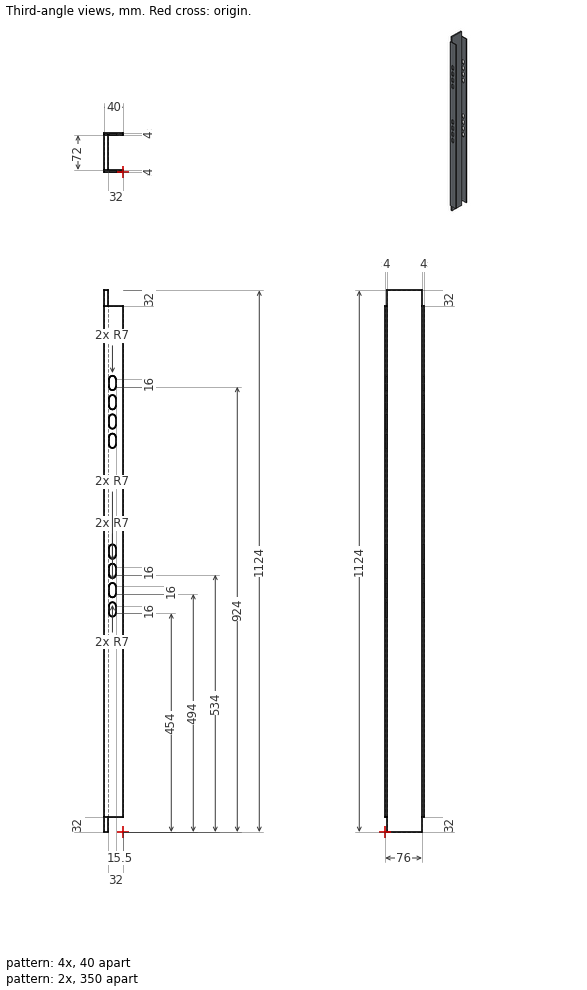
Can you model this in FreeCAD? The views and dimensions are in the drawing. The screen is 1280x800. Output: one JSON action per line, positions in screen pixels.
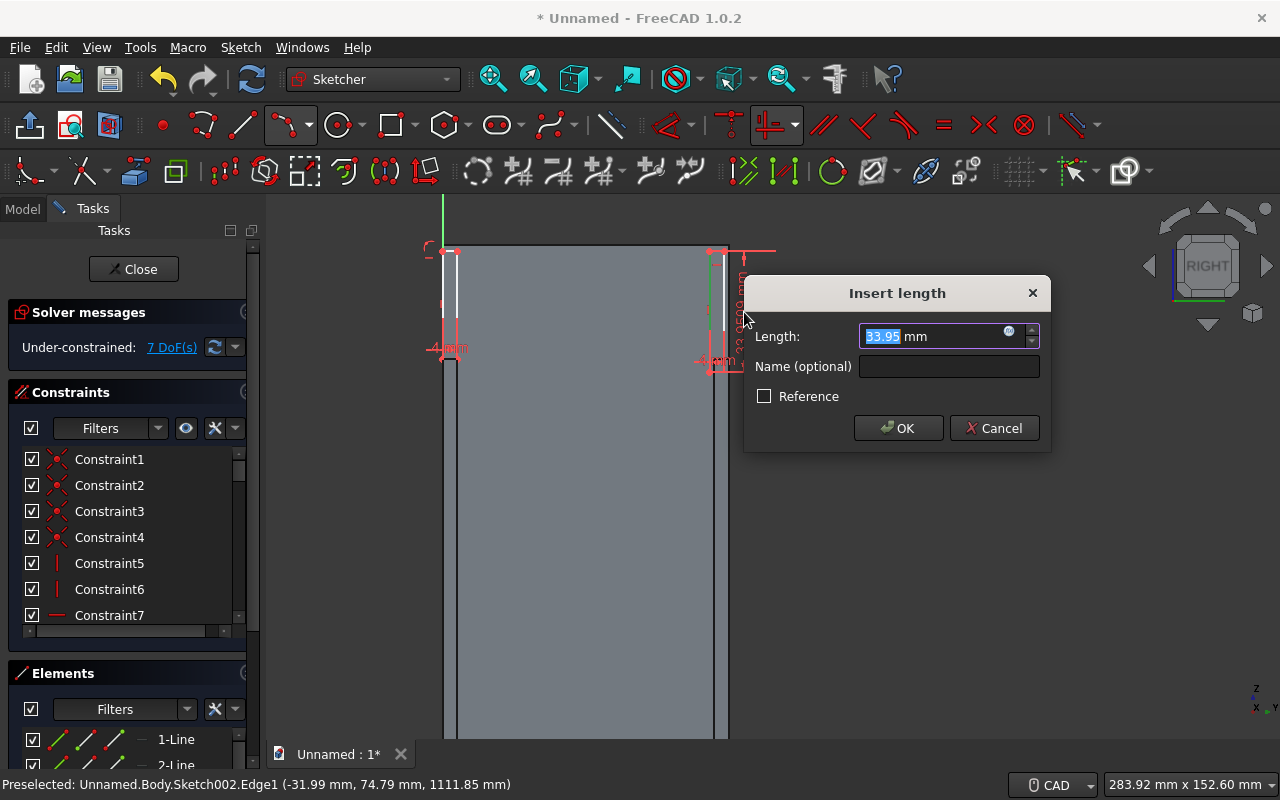
{"action": "type", "text": "32"}
{"action": "key", "text": "Return"}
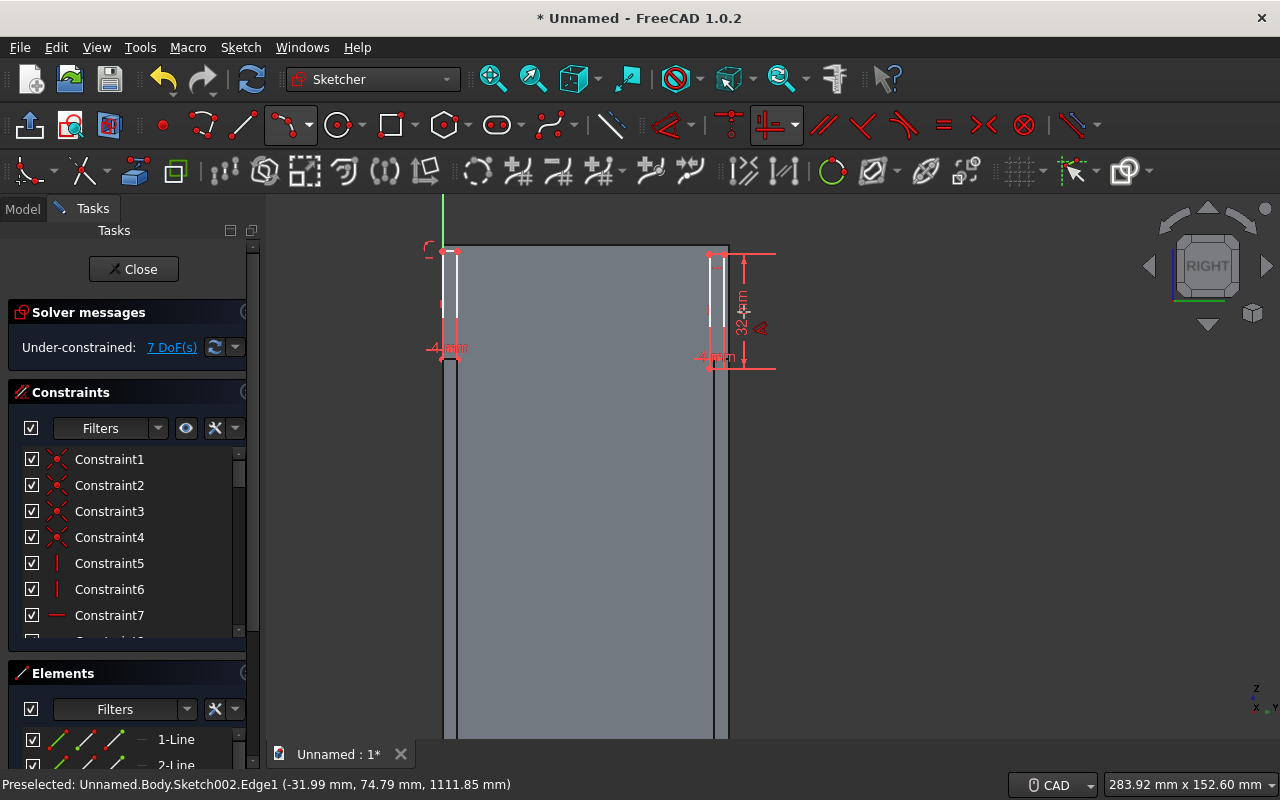
{"action": "left_click", "coordinate": [443, 284]}
{"action": "left_click", "coordinate": [409, 305]}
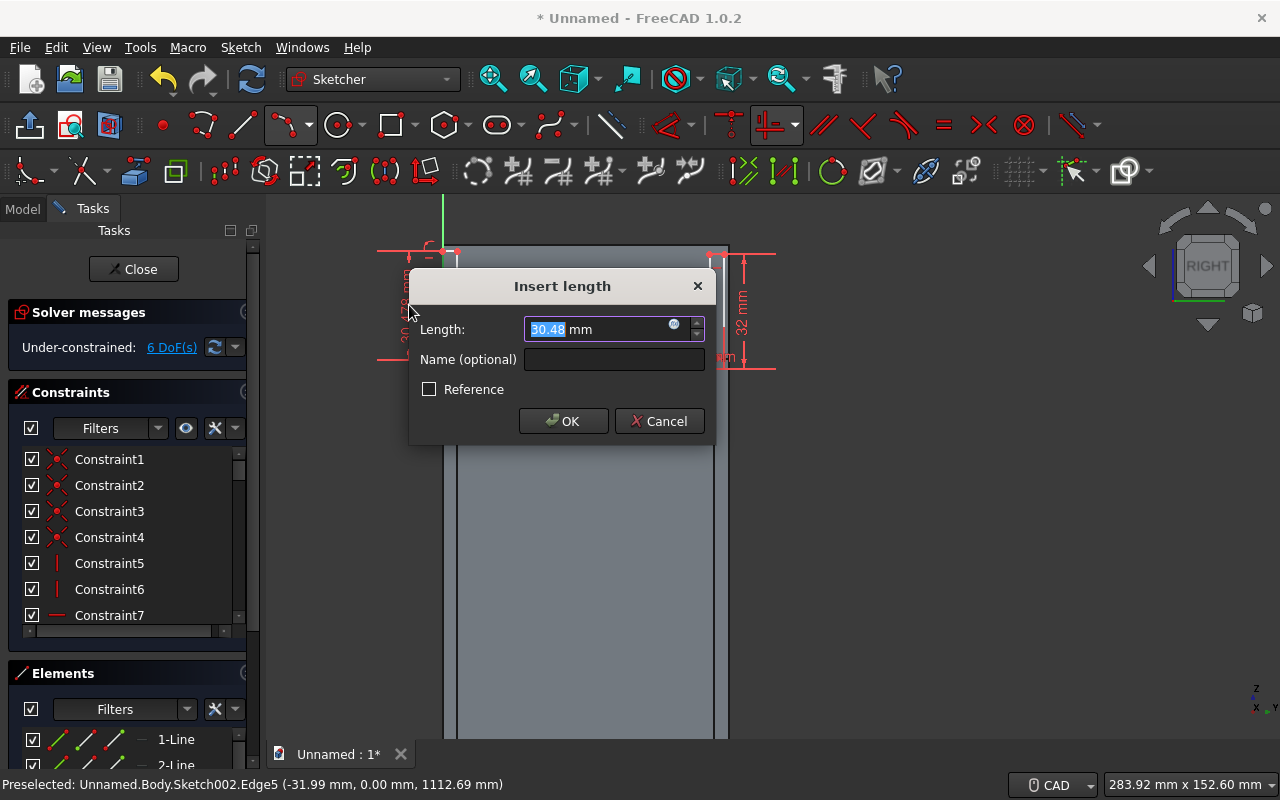
{"action": "type", "text": "32"}
{"action": "key", "text": "Return"}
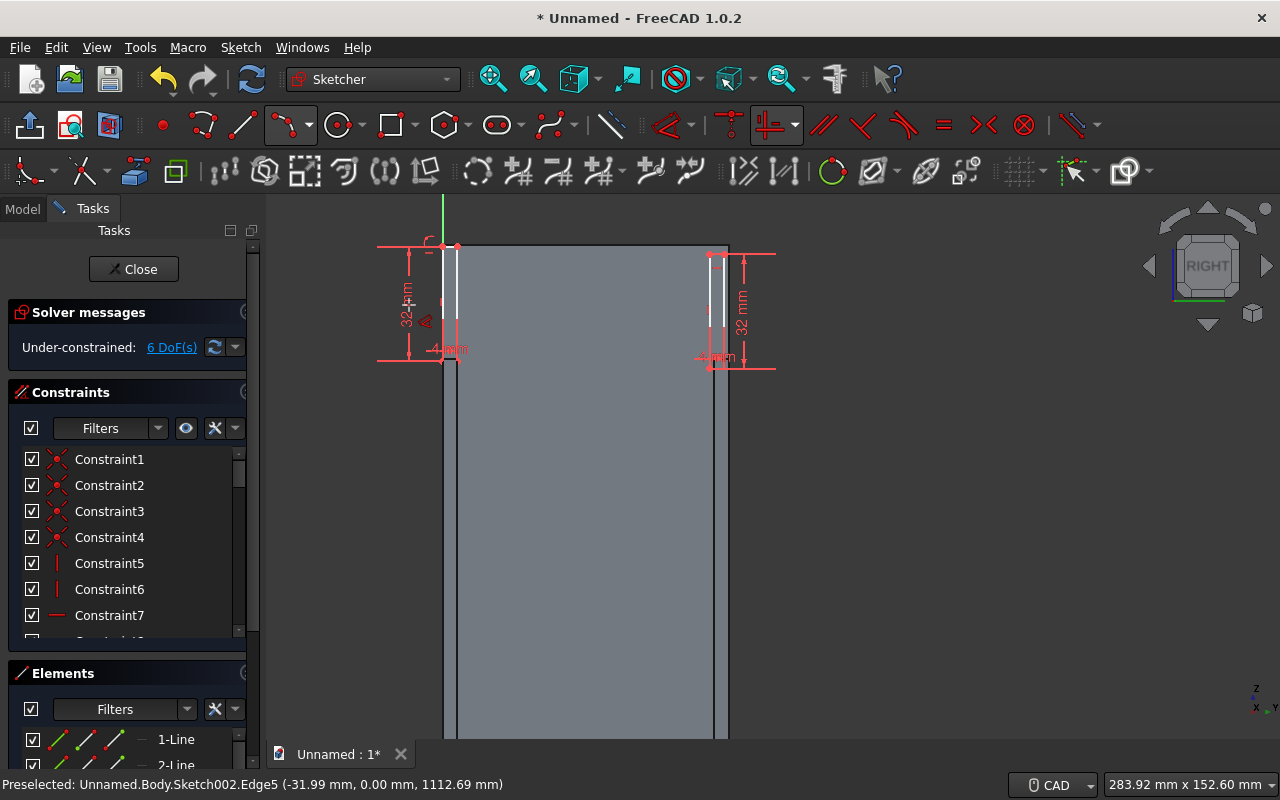
{"action": "scroll", "coordinate": [716, 288], "scroll_direction": "down", "scroll_amount": 12}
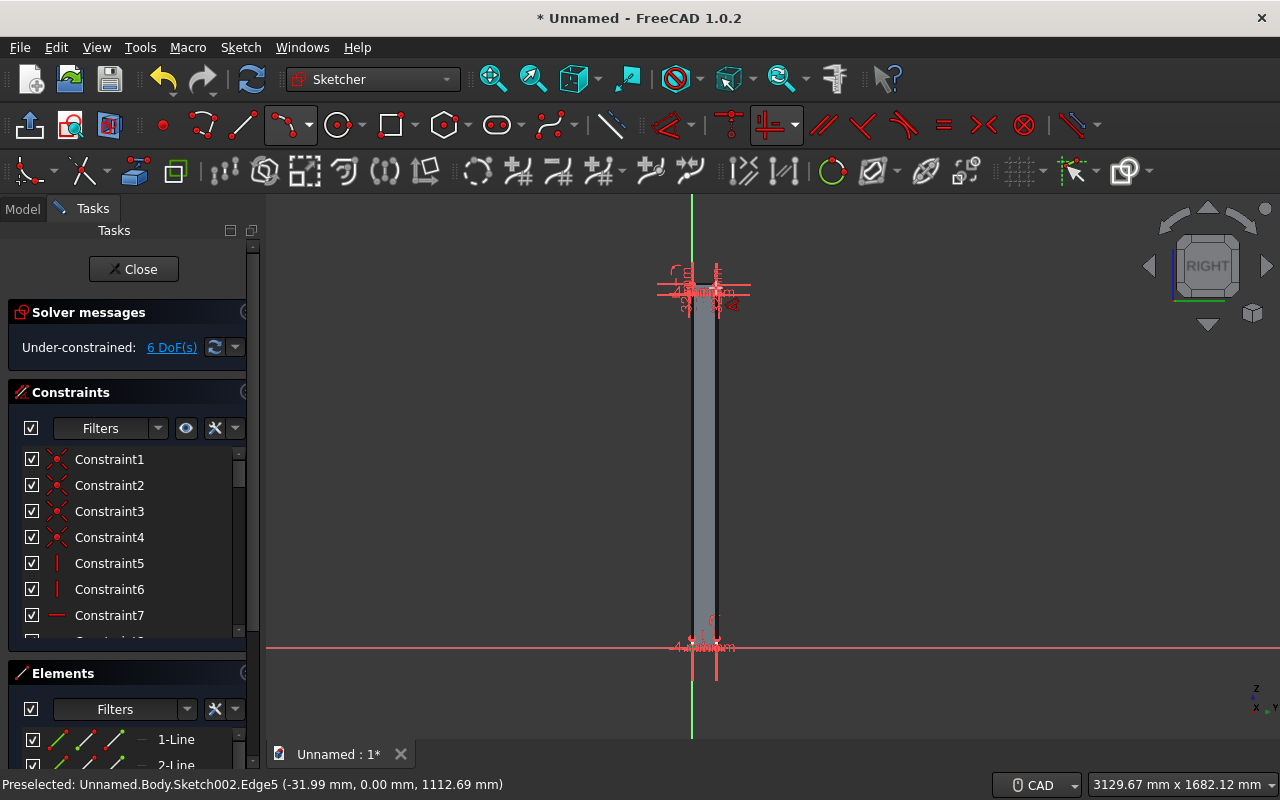
{"action": "scroll", "coordinate": [716, 642], "scroll_direction": "up", "scroll_amount": 12}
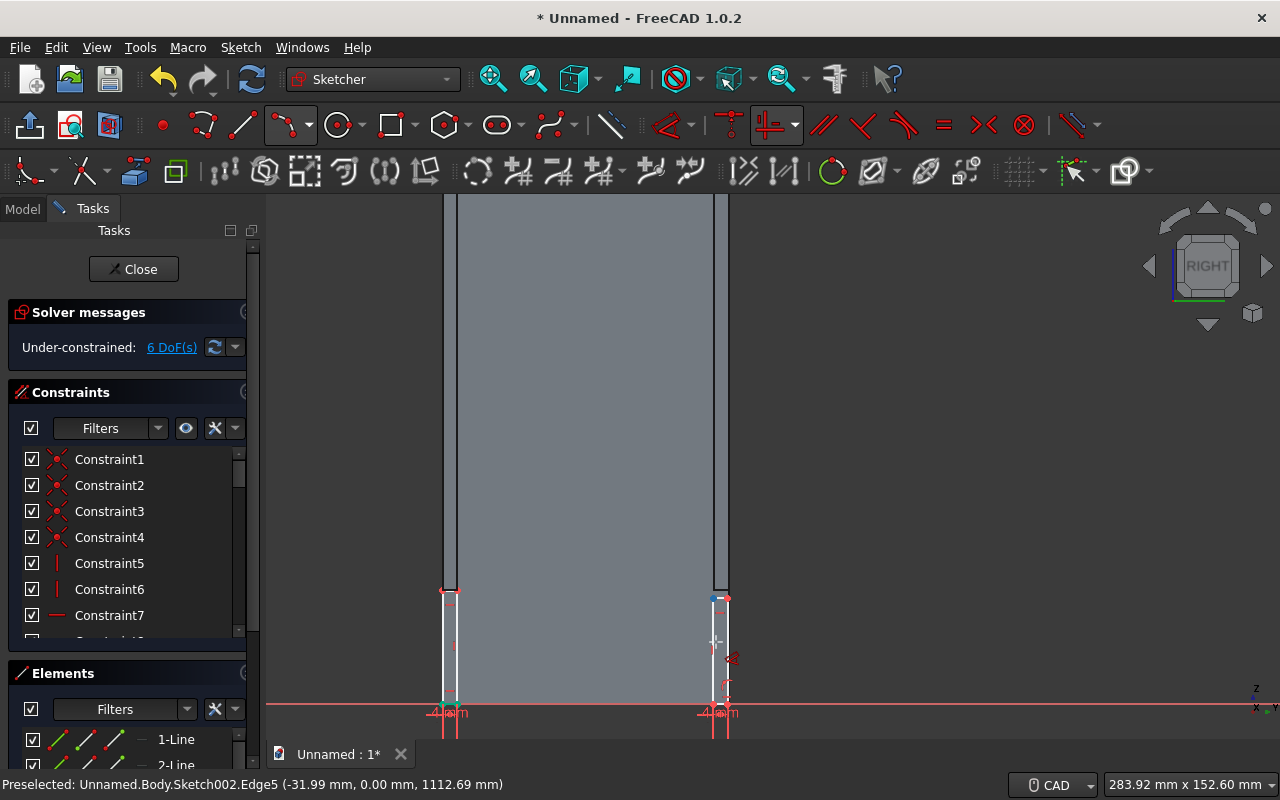
{"action": "left_click", "coordinate": [713, 630]}
{"action": "left_click", "coordinate": [747, 651]}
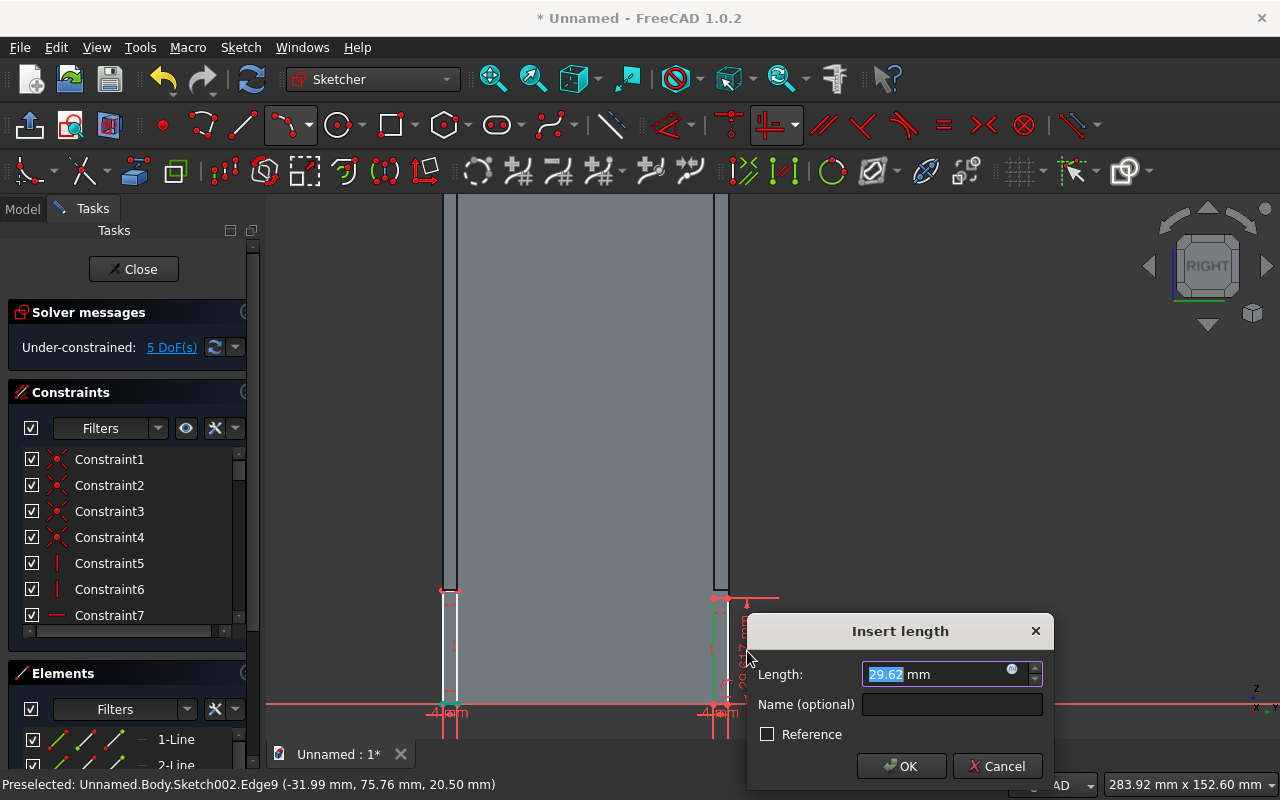
{"action": "type", "text": "32"}
{"action": "key", "text": "Return"}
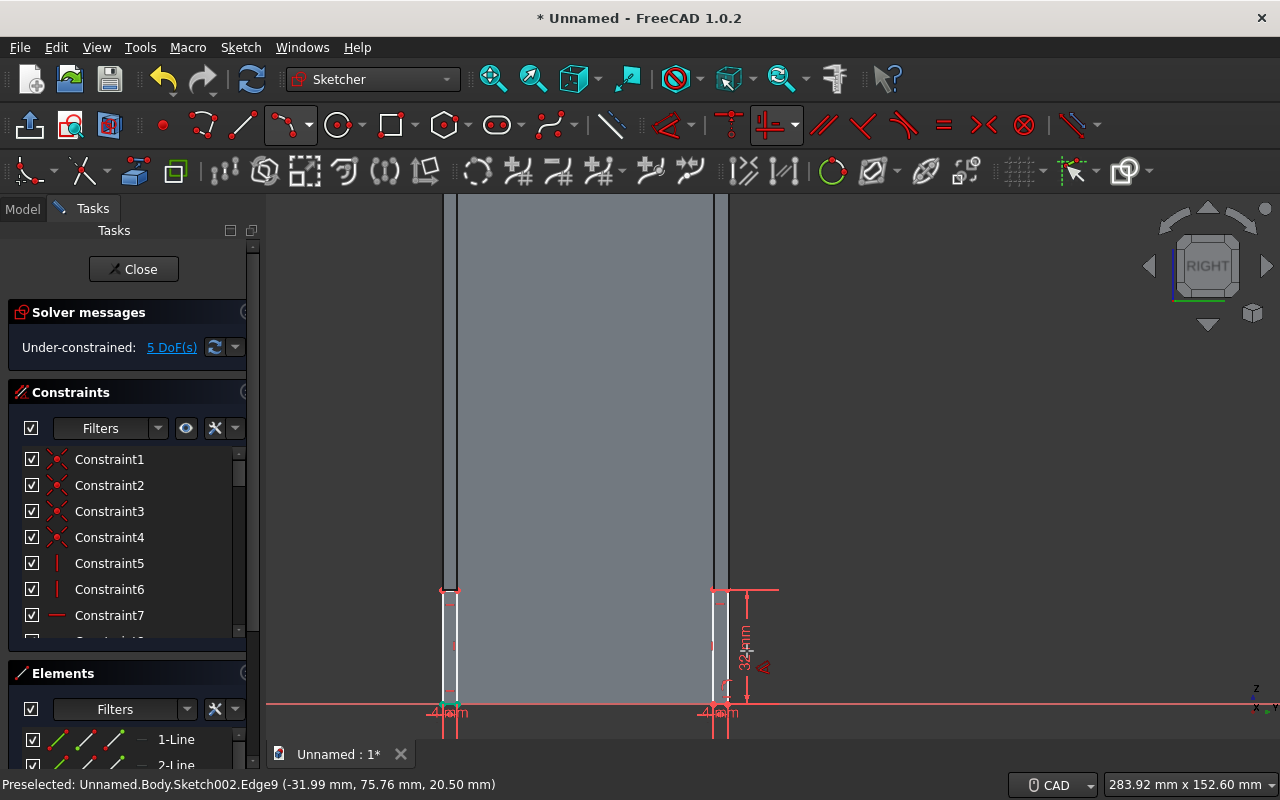
{"action": "left_click", "coordinate": [457, 670]}
{"action": "left_click", "coordinate": [423, 647]}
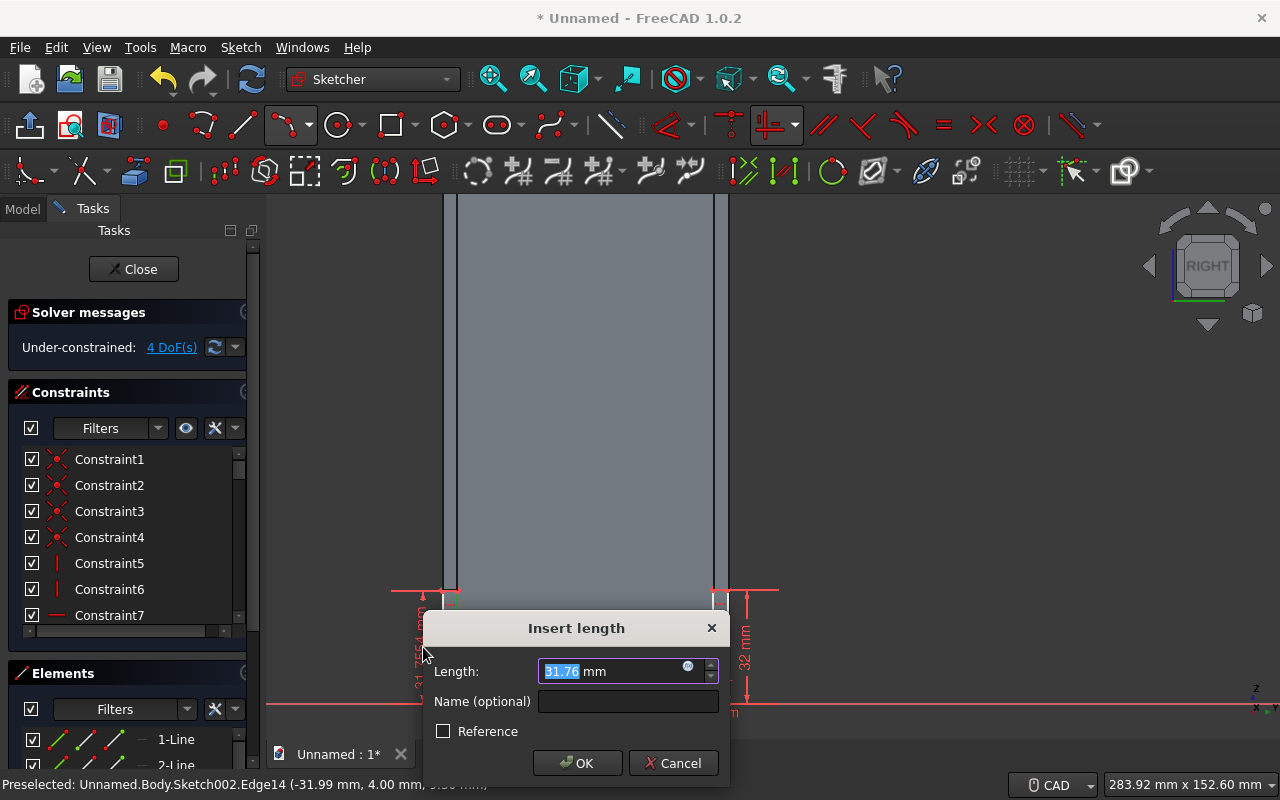
{"action": "type", "text": "32"}
{"action": "key", "text": "Return"}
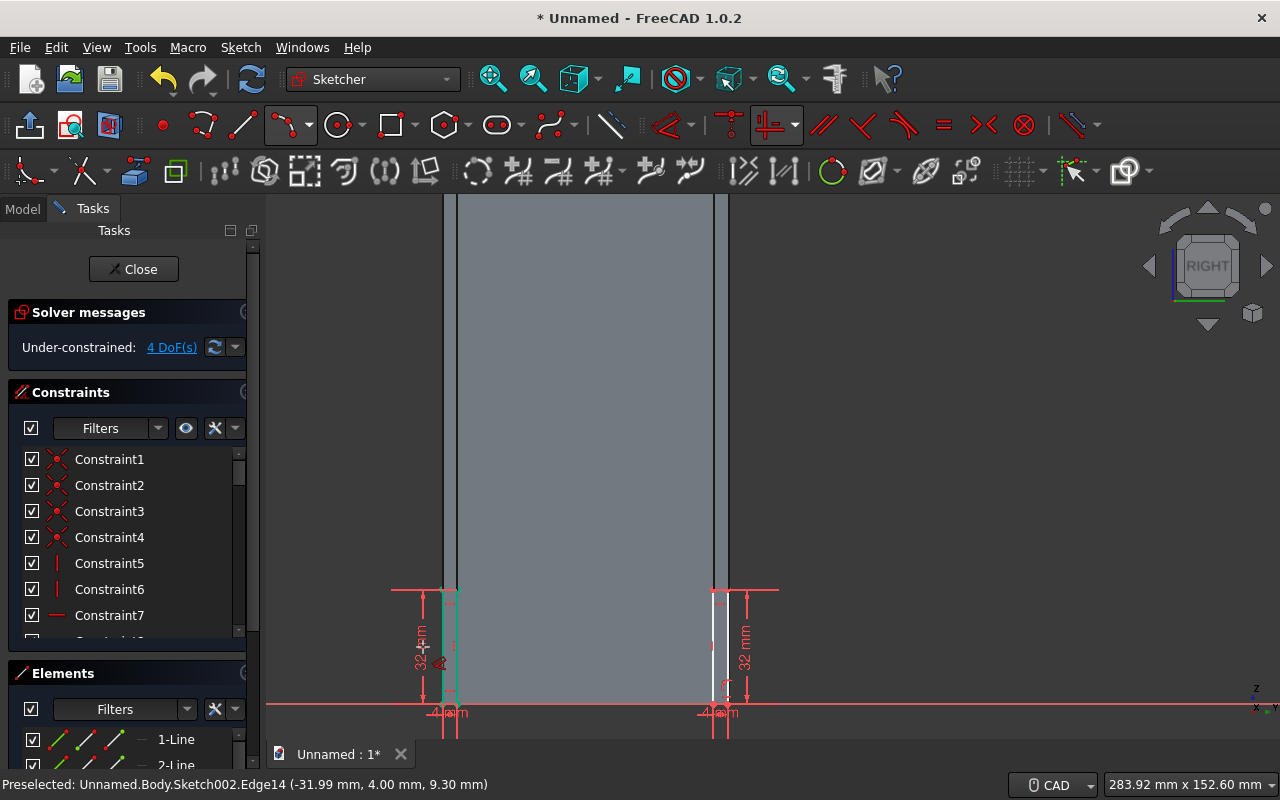
{"action": "scroll", "coordinate": [716, 643], "scroll_direction": "down", "scroll_amount": 12}